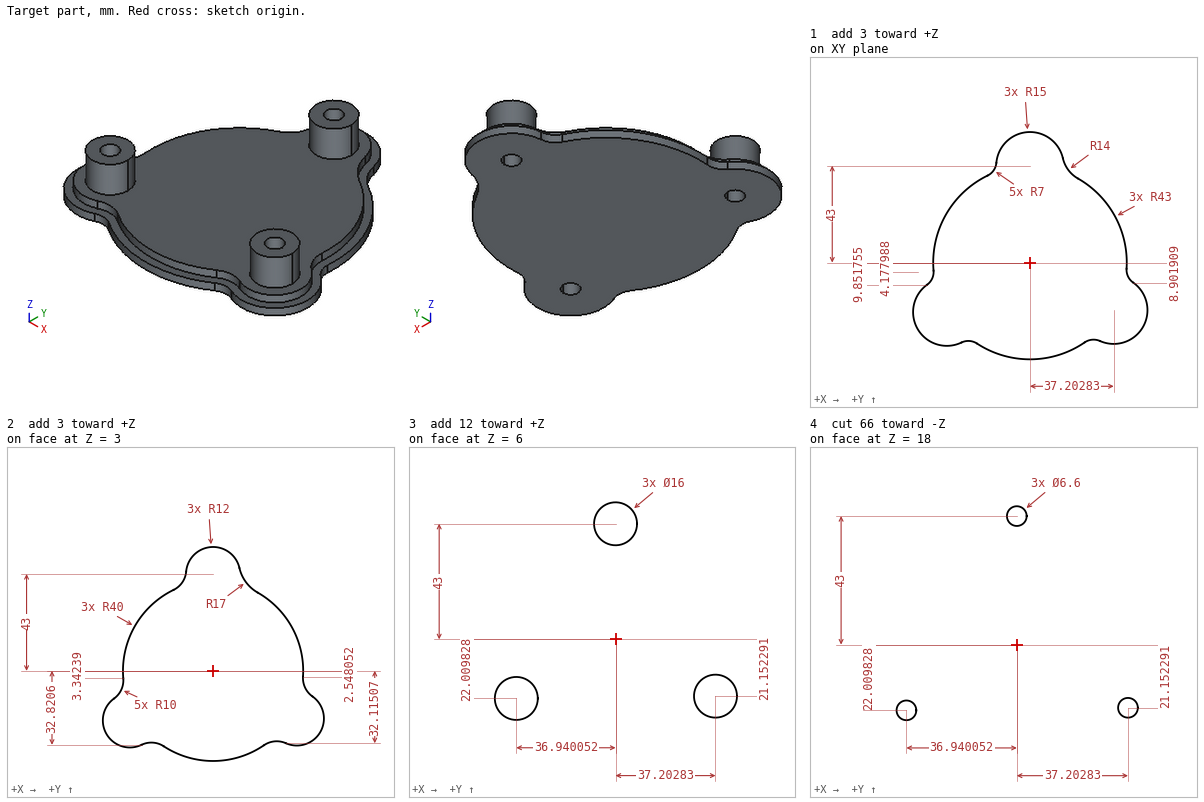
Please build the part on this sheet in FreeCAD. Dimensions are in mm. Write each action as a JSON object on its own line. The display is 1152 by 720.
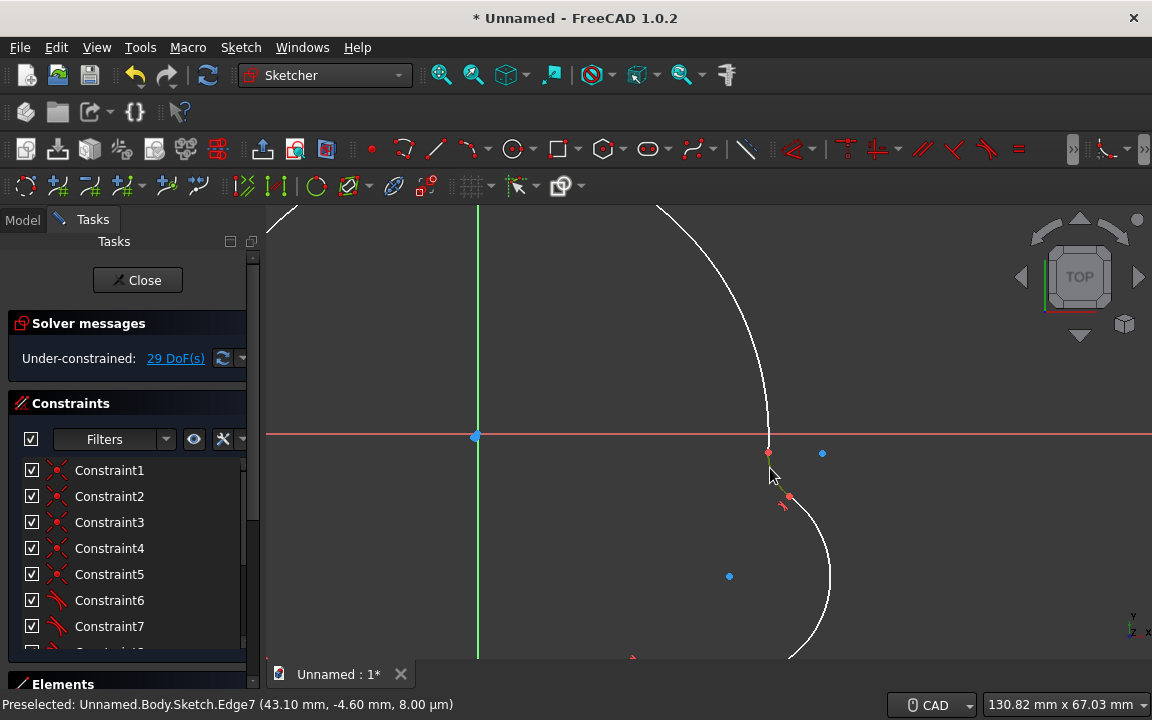
{"action": "left_click", "coordinate": [758, 357]}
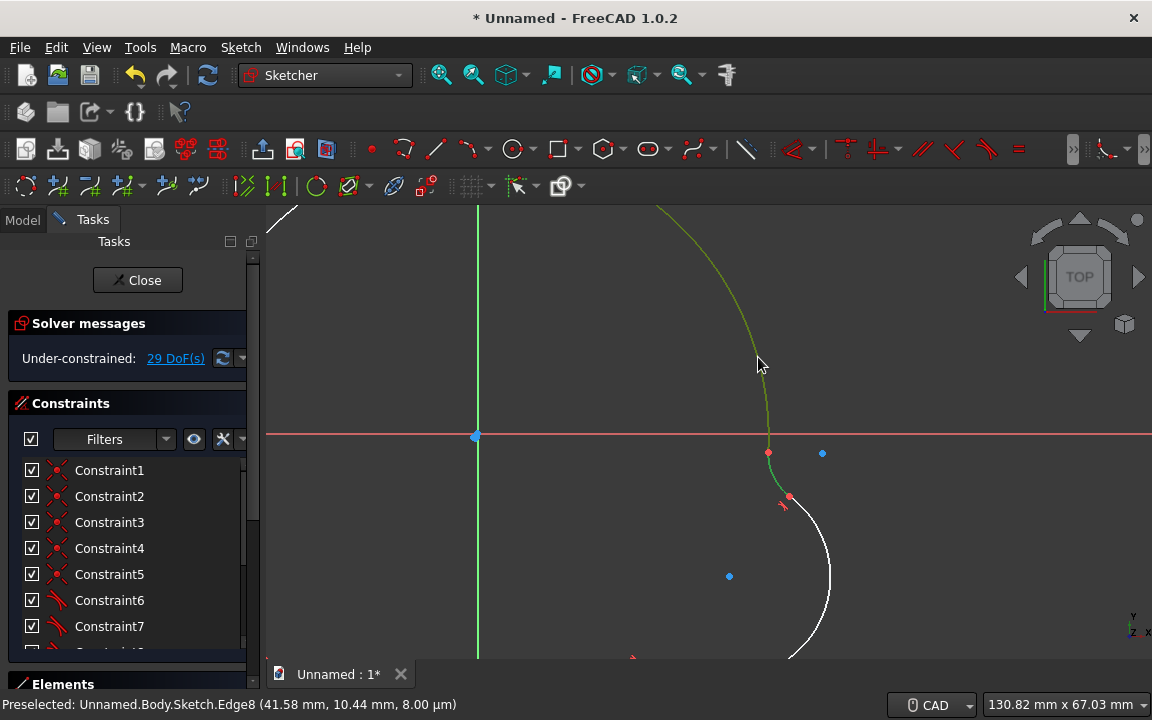
{"action": "left_click", "coordinate": [988, 150]}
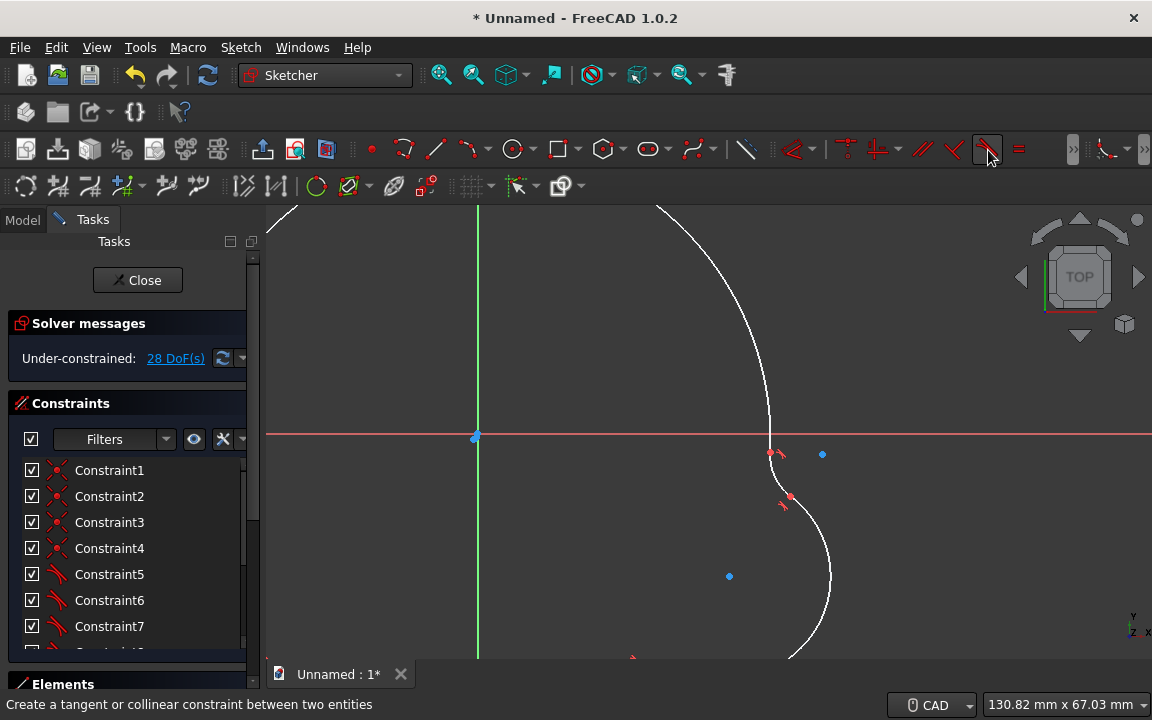
{"action": "left_click", "coordinate": [759, 356]}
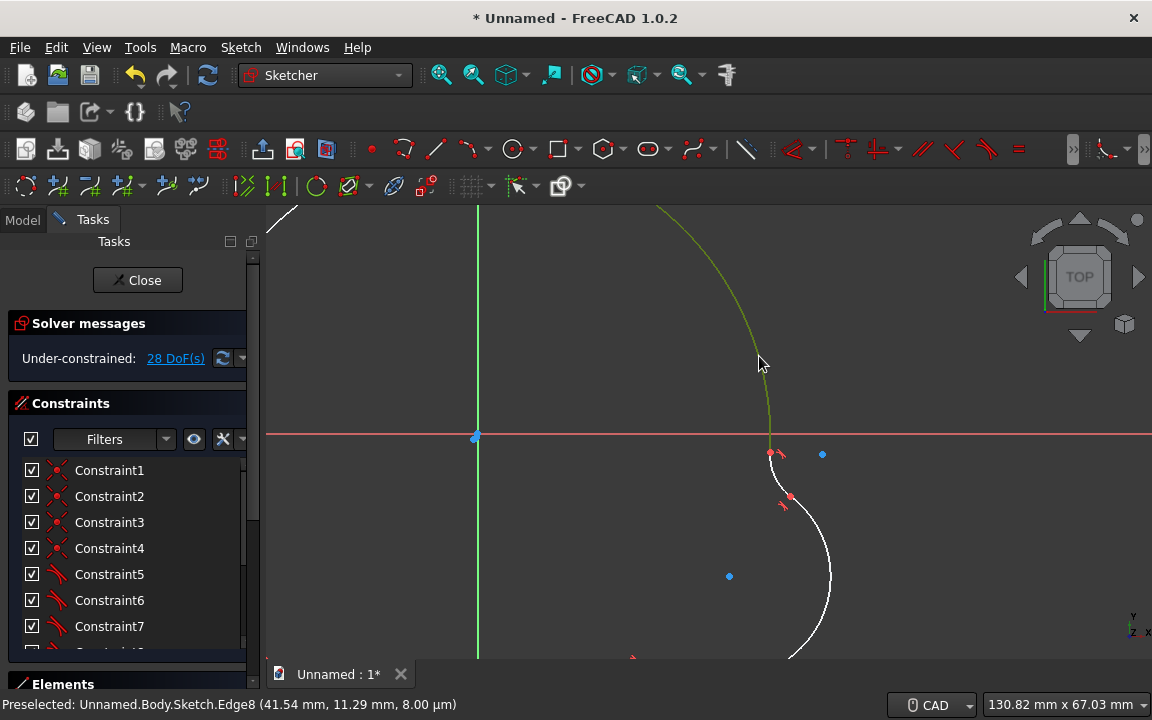
{"action": "scroll", "coordinate": [772, 472], "scroll_direction": "down", "scroll_amount": 4}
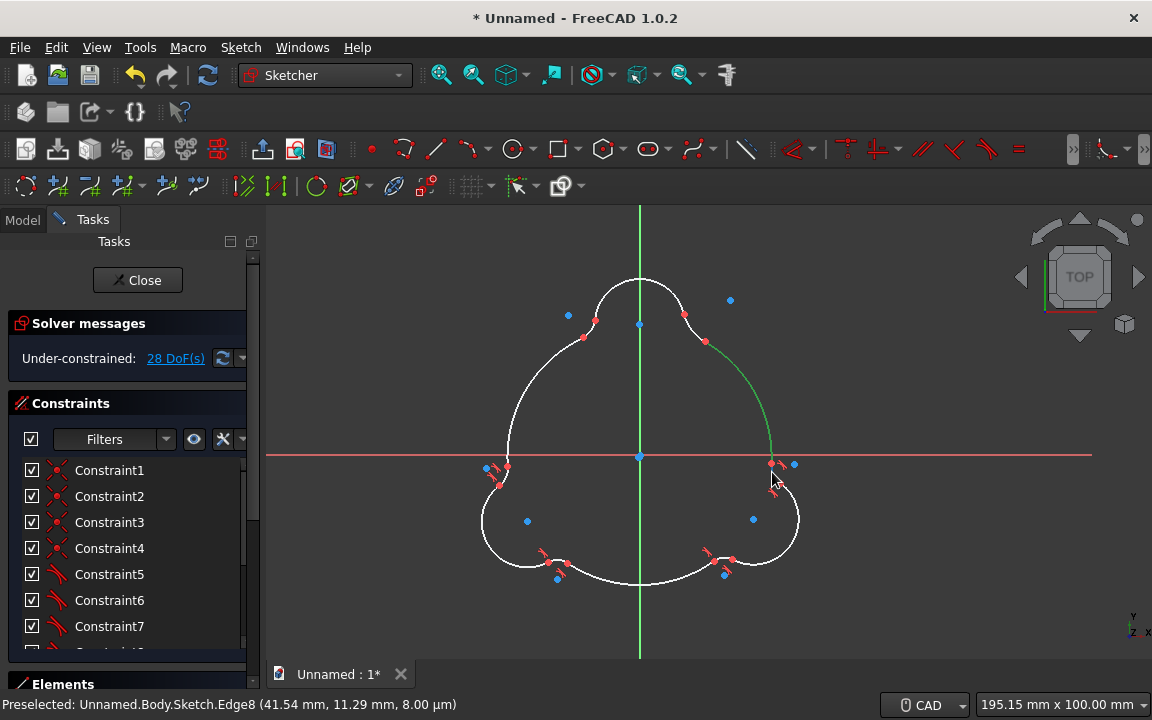
{"action": "scroll", "coordinate": [688, 325], "scroll_direction": "up", "scroll_amount": 2}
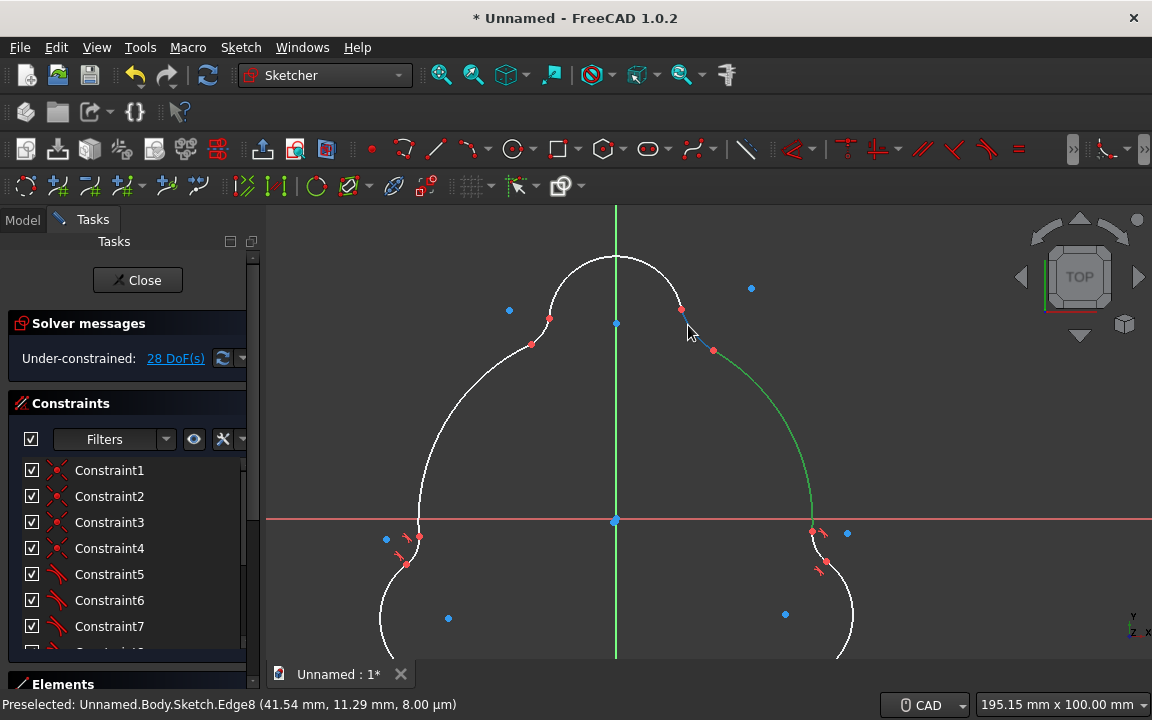
{"action": "left_click", "coordinate": [688, 324]}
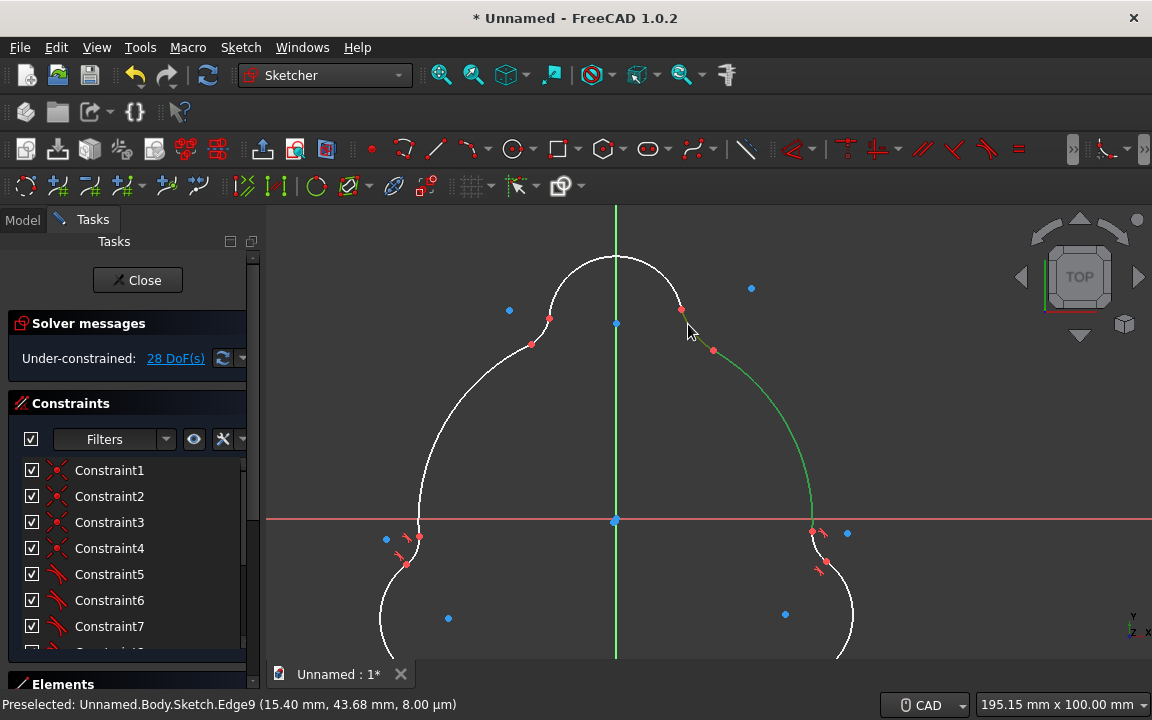
{"action": "left_click", "coordinate": [988, 150]}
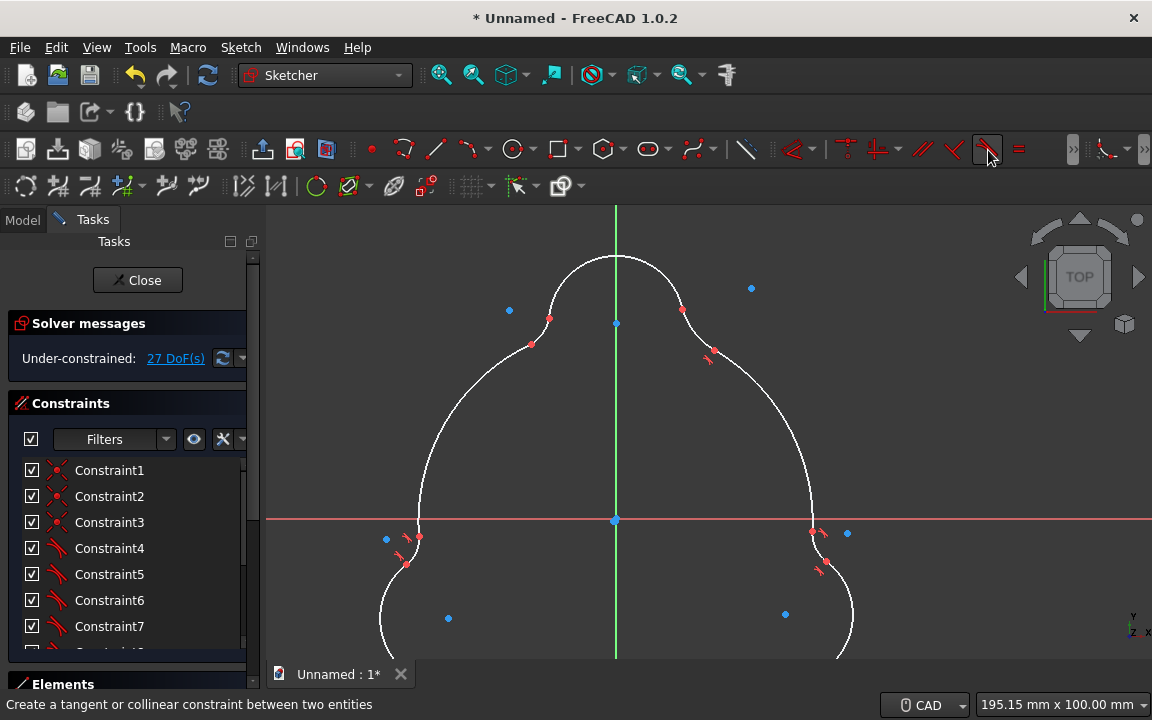
{"action": "left_click", "coordinate": [689, 324]}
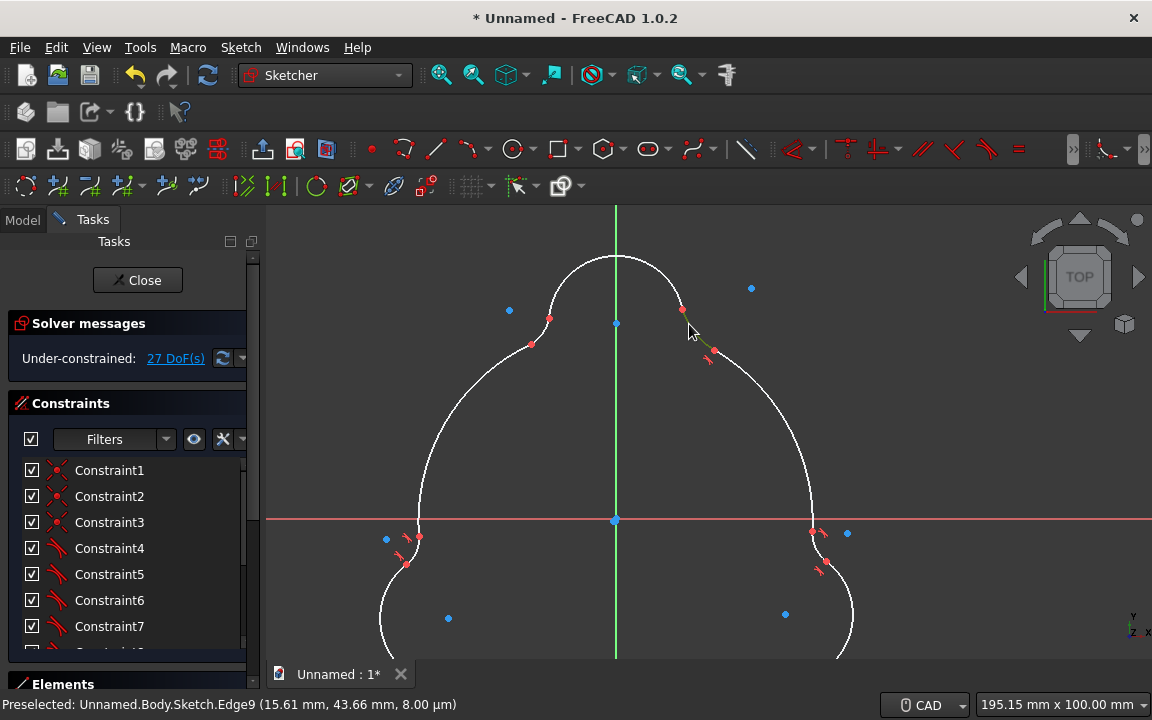
{"action": "left_click", "coordinate": [649, 264]}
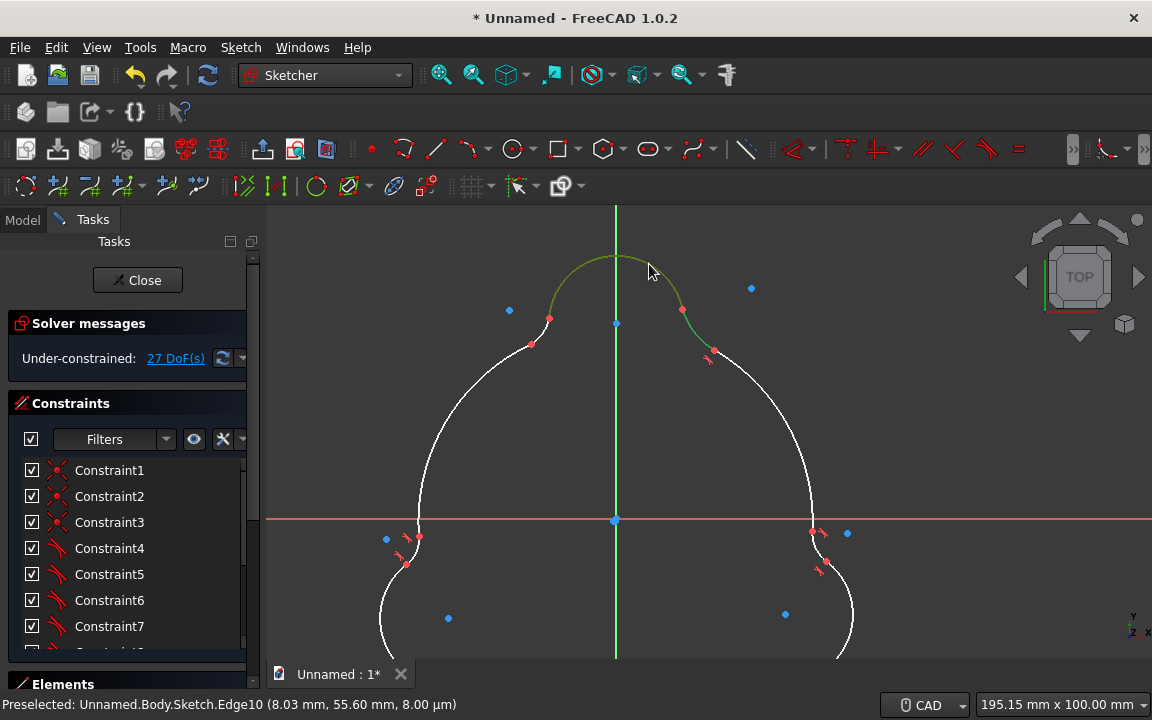
{"action": "left_click", "coordinate": [988, 150]}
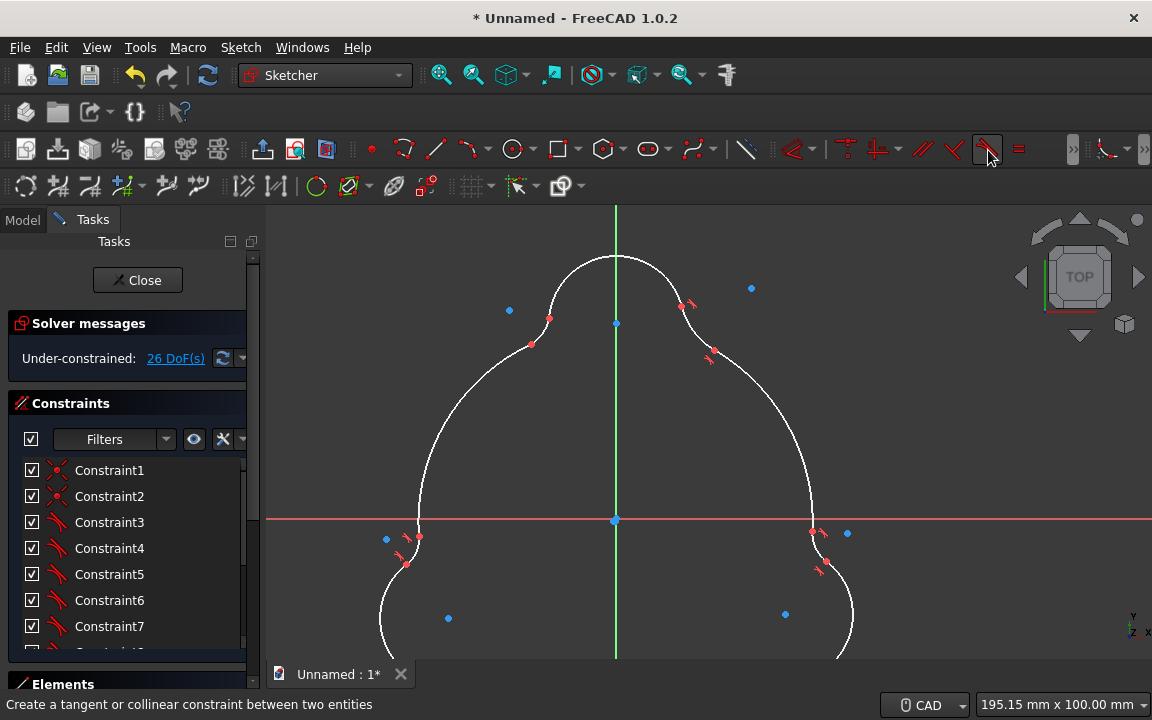
{"action": "left_click", "coordinate": [647, 263]}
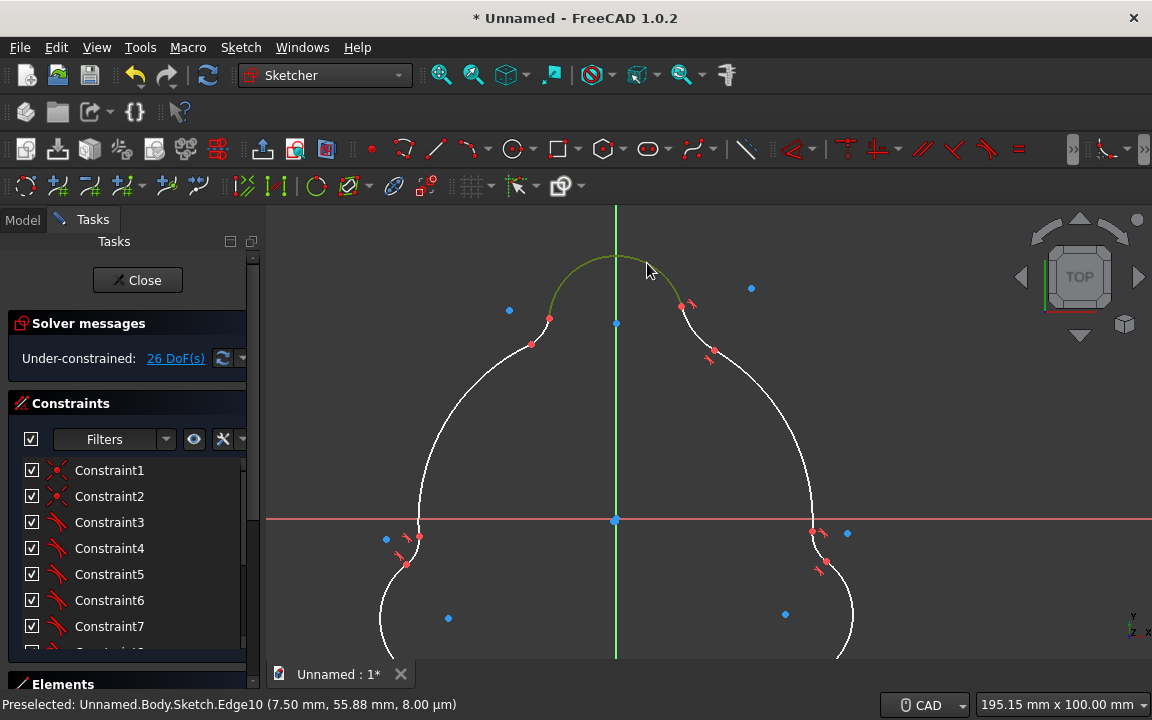
{"action": "scroll", "coordinate": [539, 338], "scroll_direction": "up", "scroll_amount": 2}